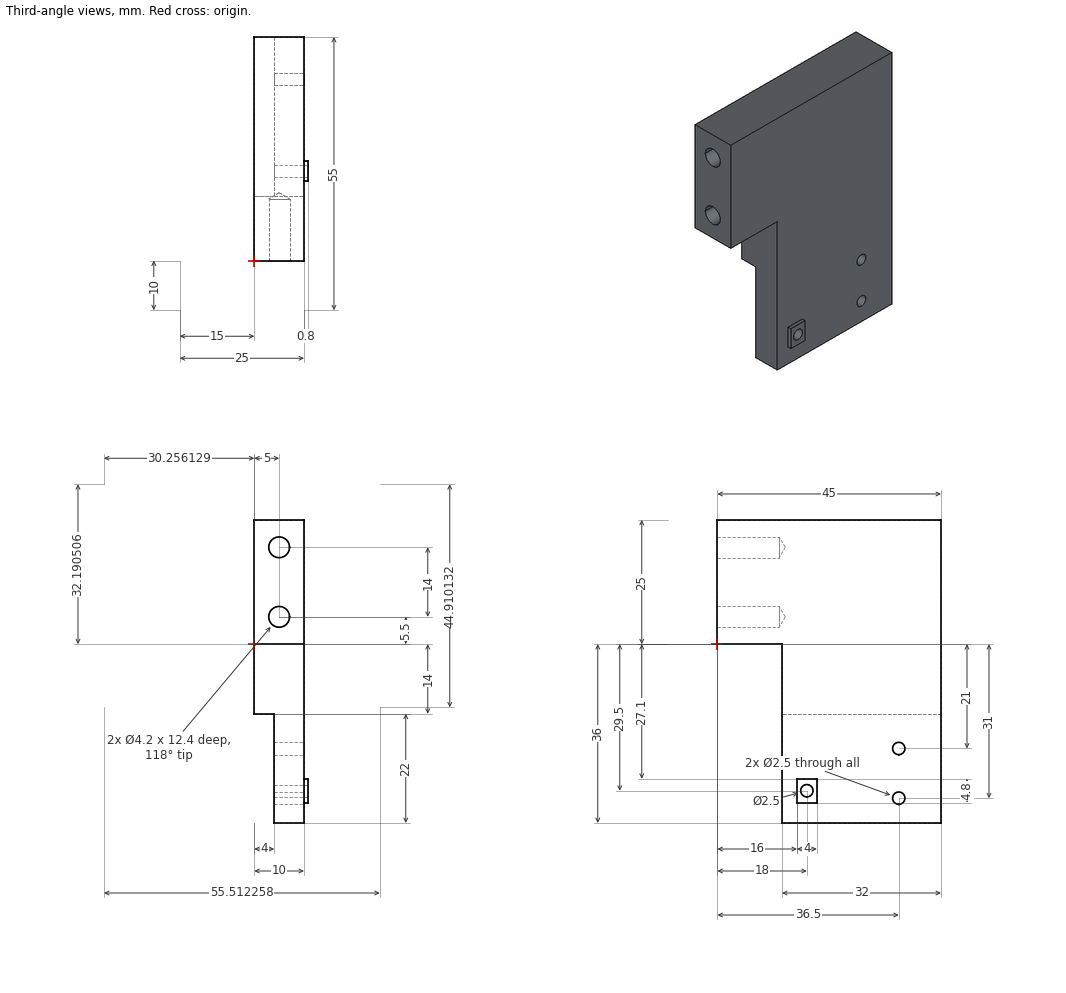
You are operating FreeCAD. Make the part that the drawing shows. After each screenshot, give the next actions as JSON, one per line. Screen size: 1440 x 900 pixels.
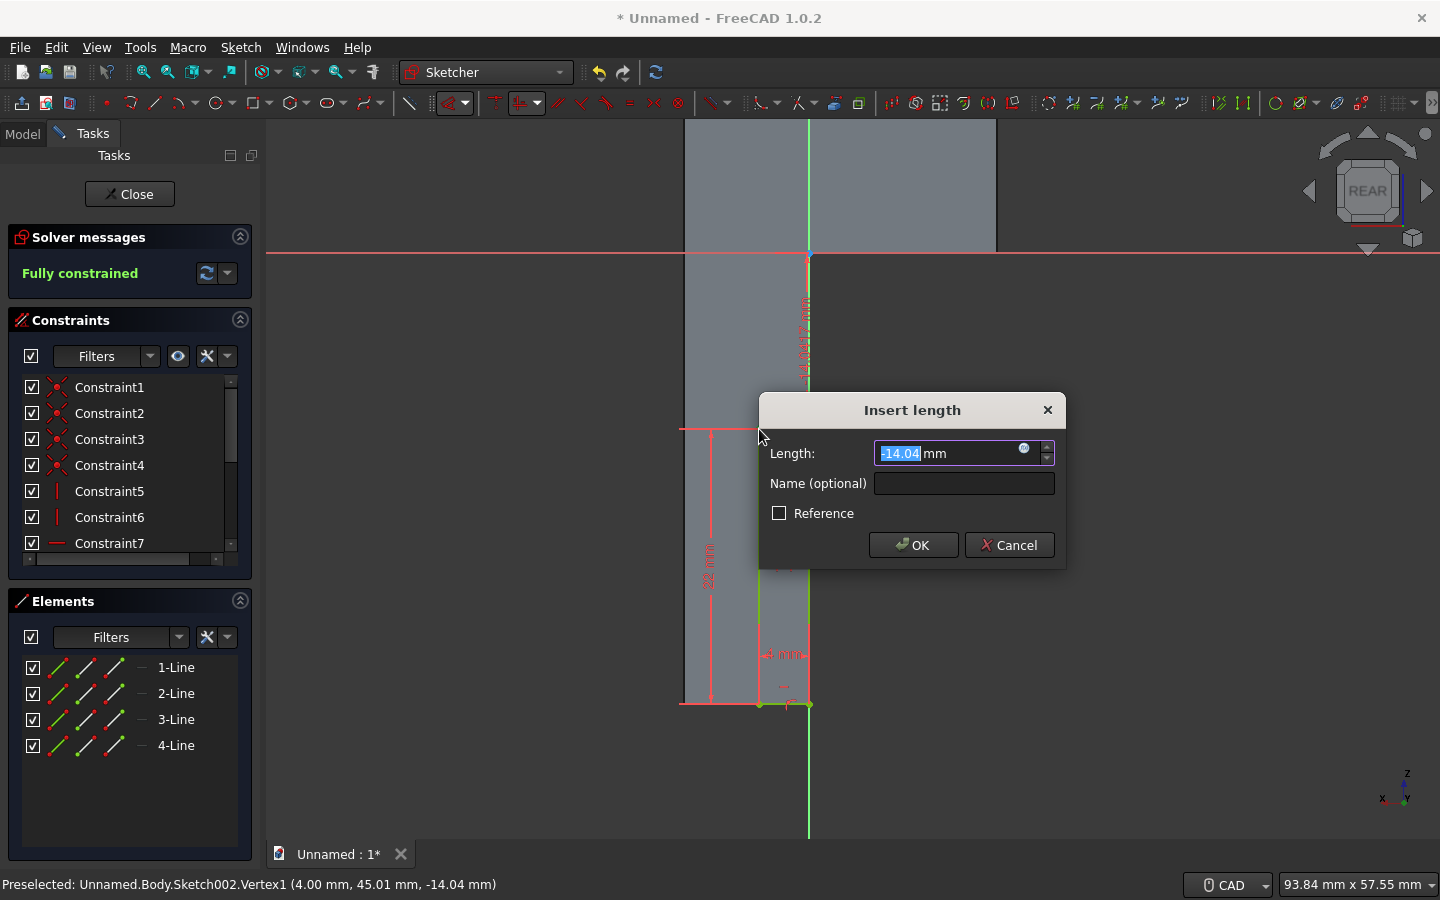
{"action": "type", "text": "-14"}
{"action": "key", "text": "Return"}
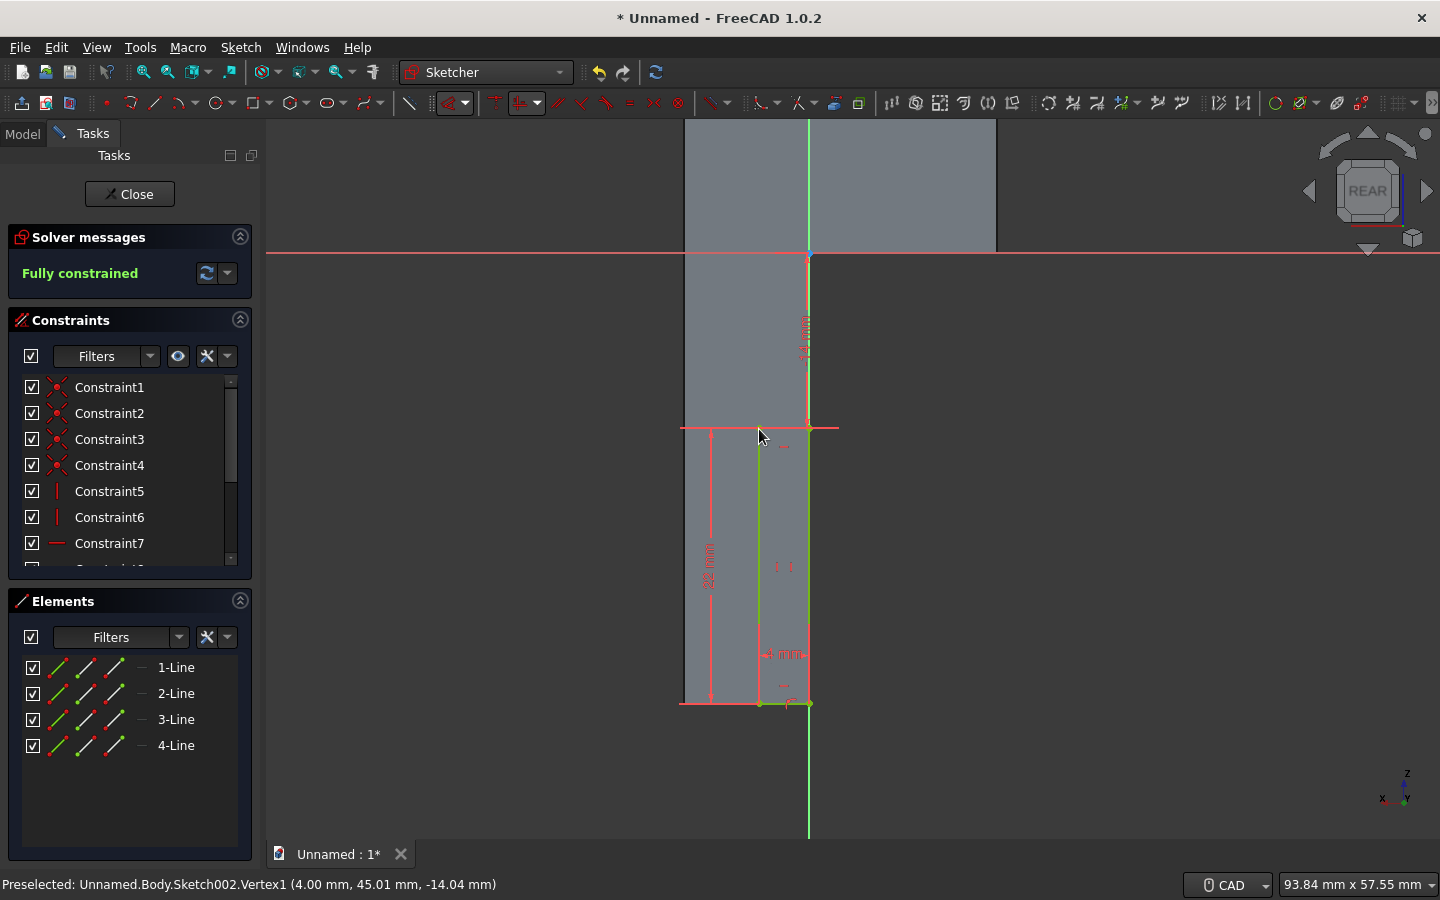
{"action": "left_click", "coordinate": [130, 194]}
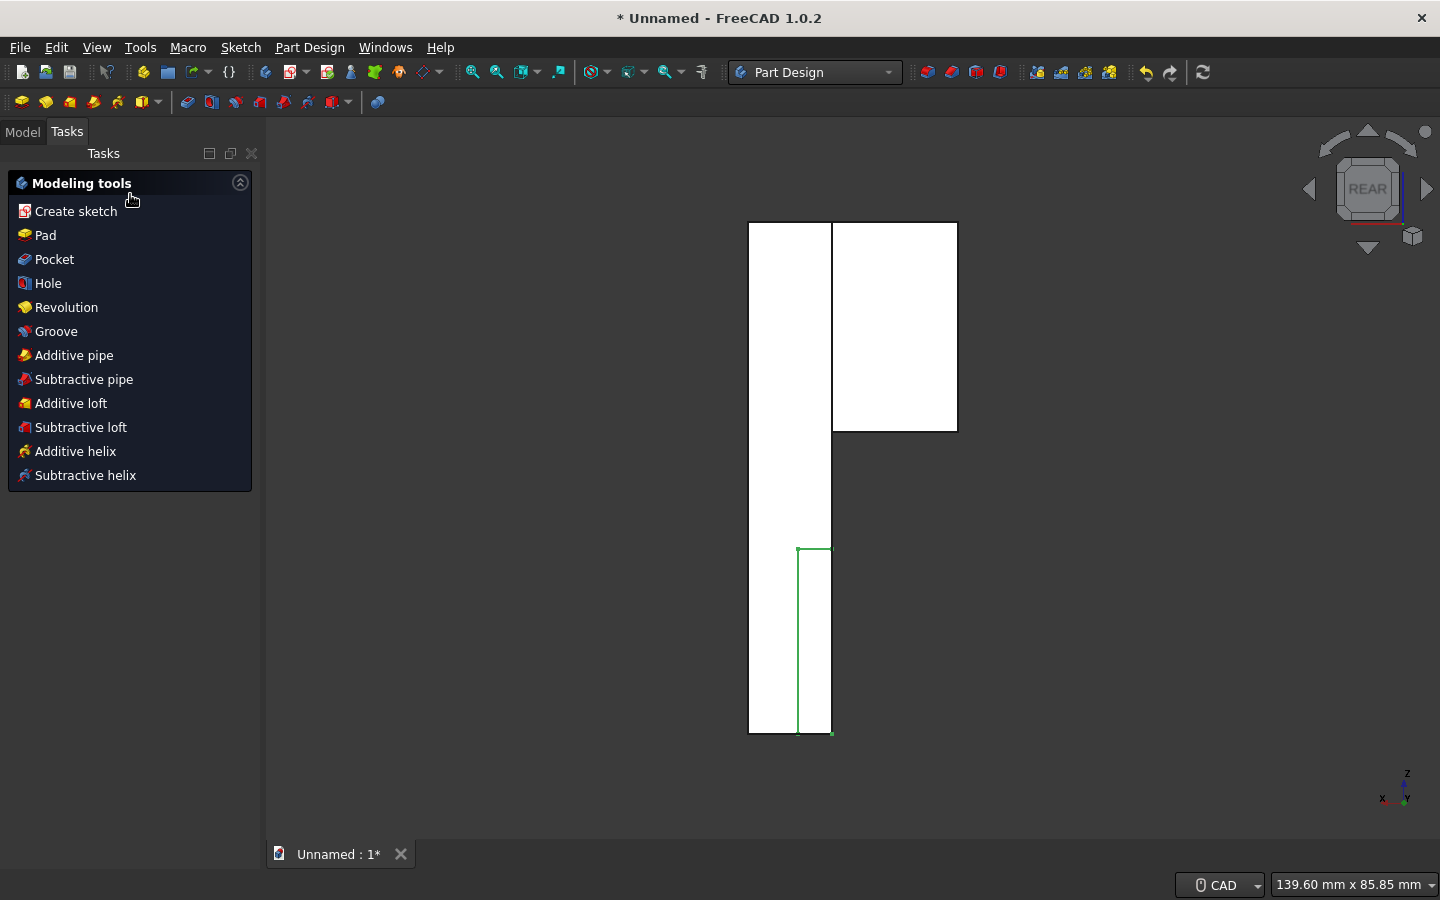
{"action": "left_click", "coordinate": [188, 102]}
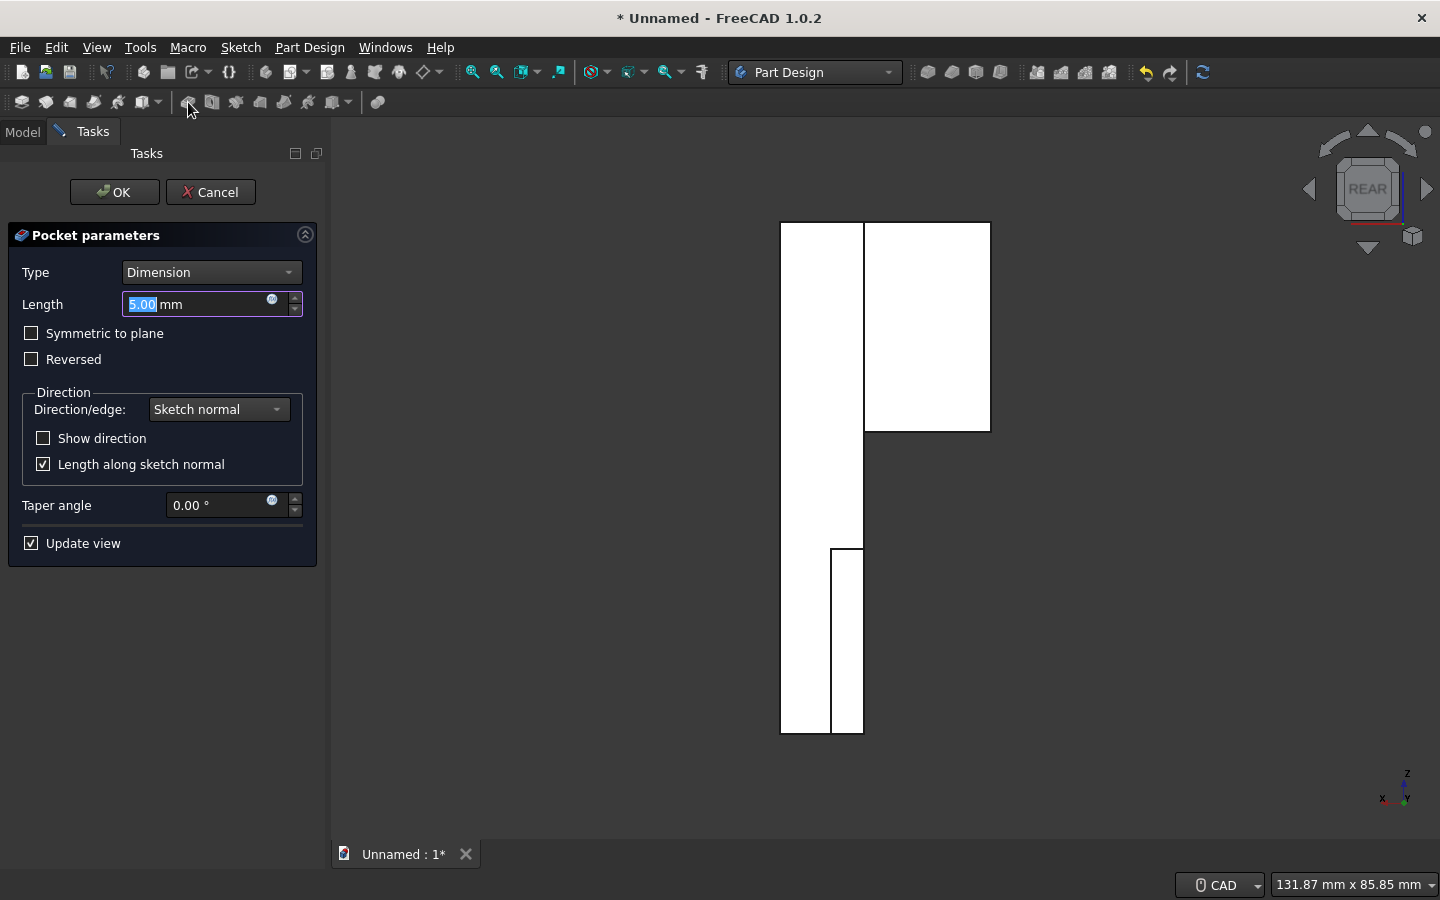
{"action": "left_click", "coordinate": [212, 272]}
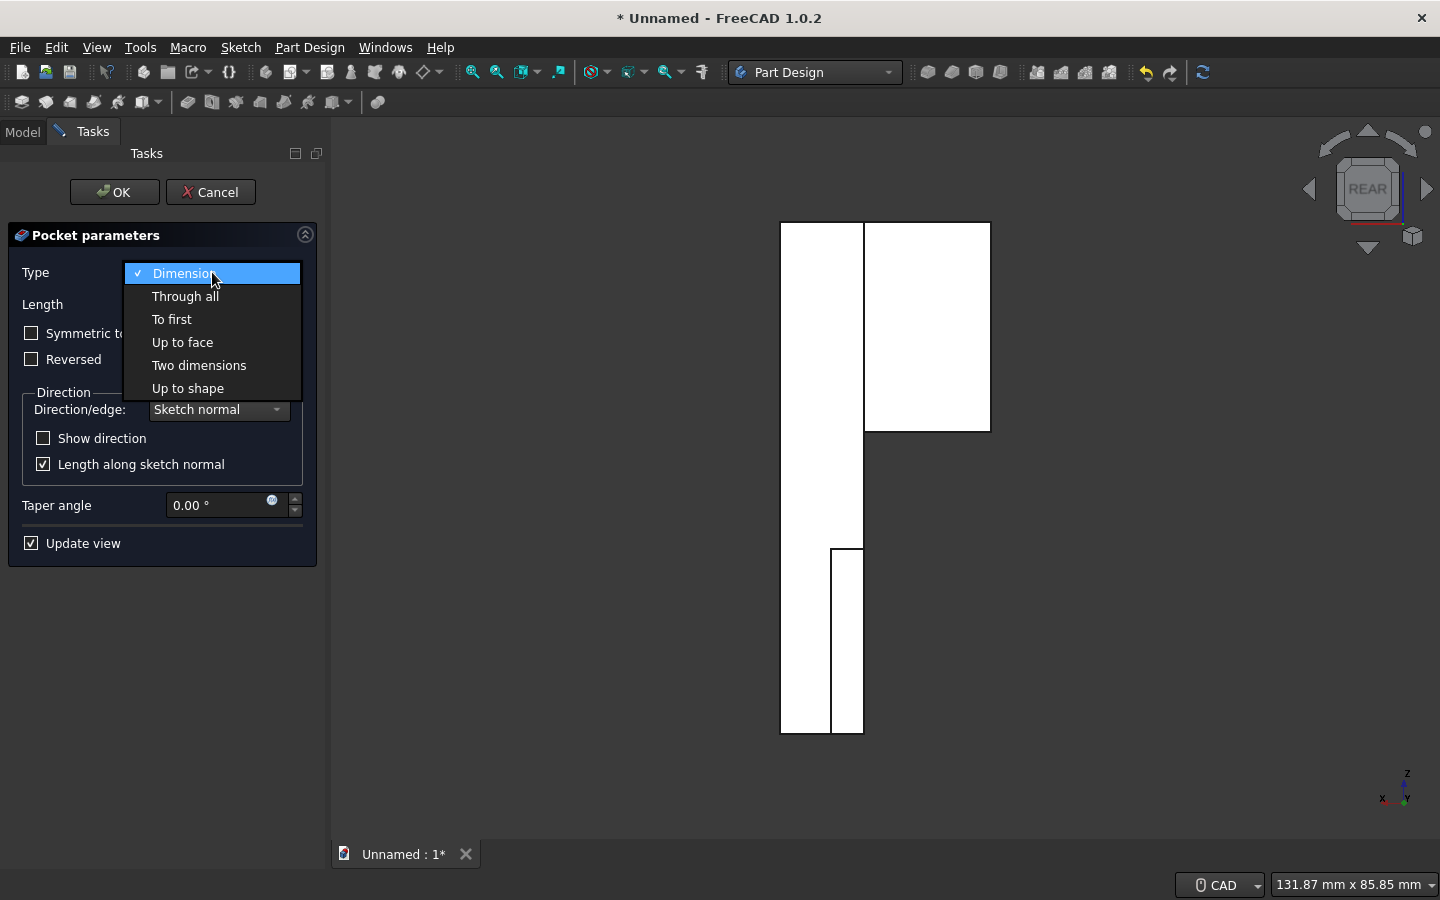
{"action": "left_click", "coordinate": [212, 296]}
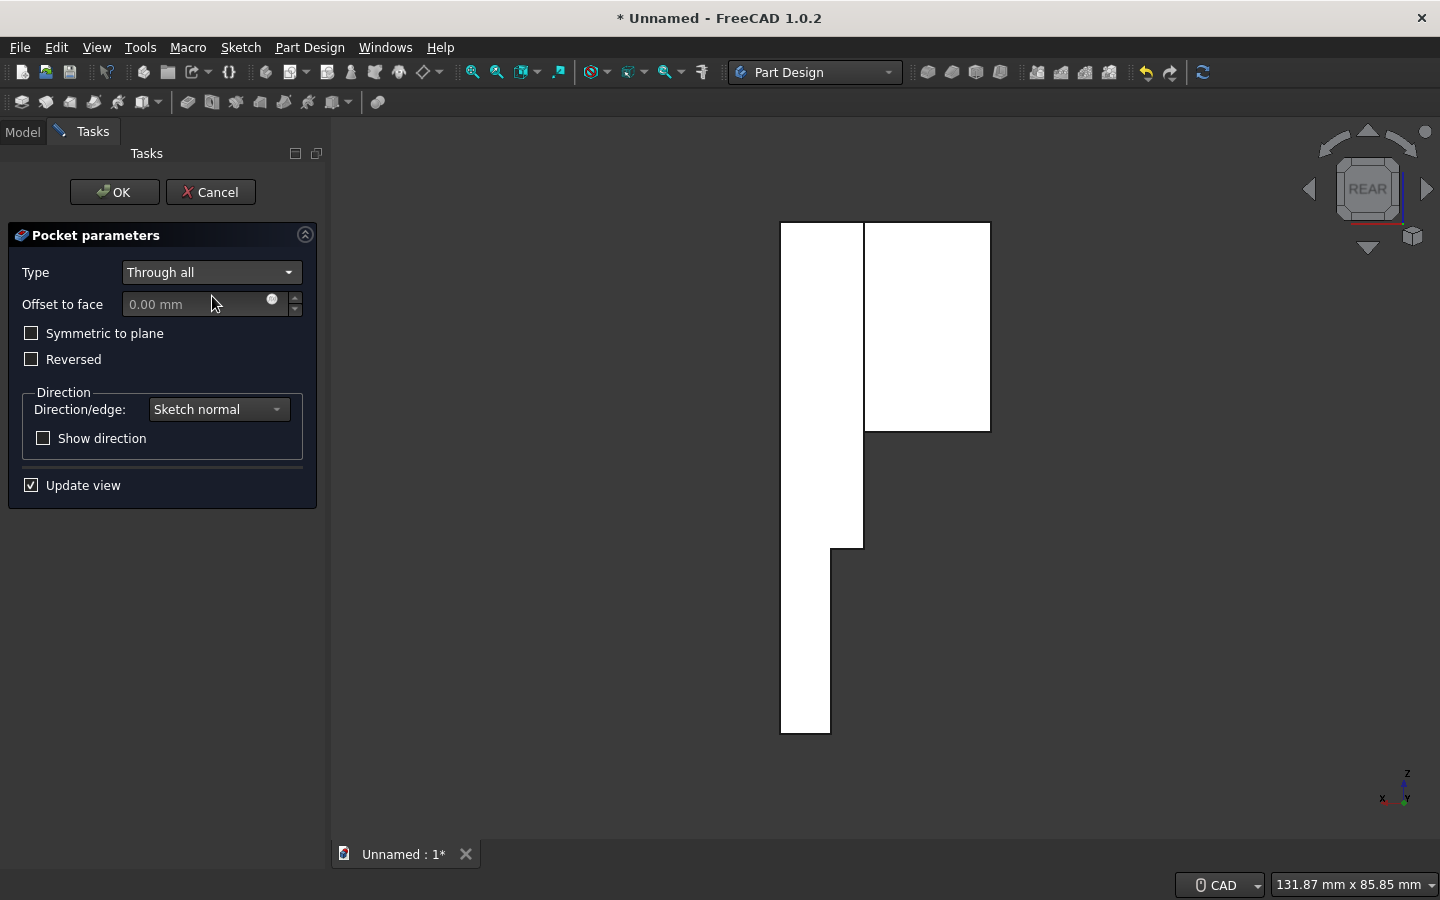
{"action": "left_click", "coordinate": [115, 192]}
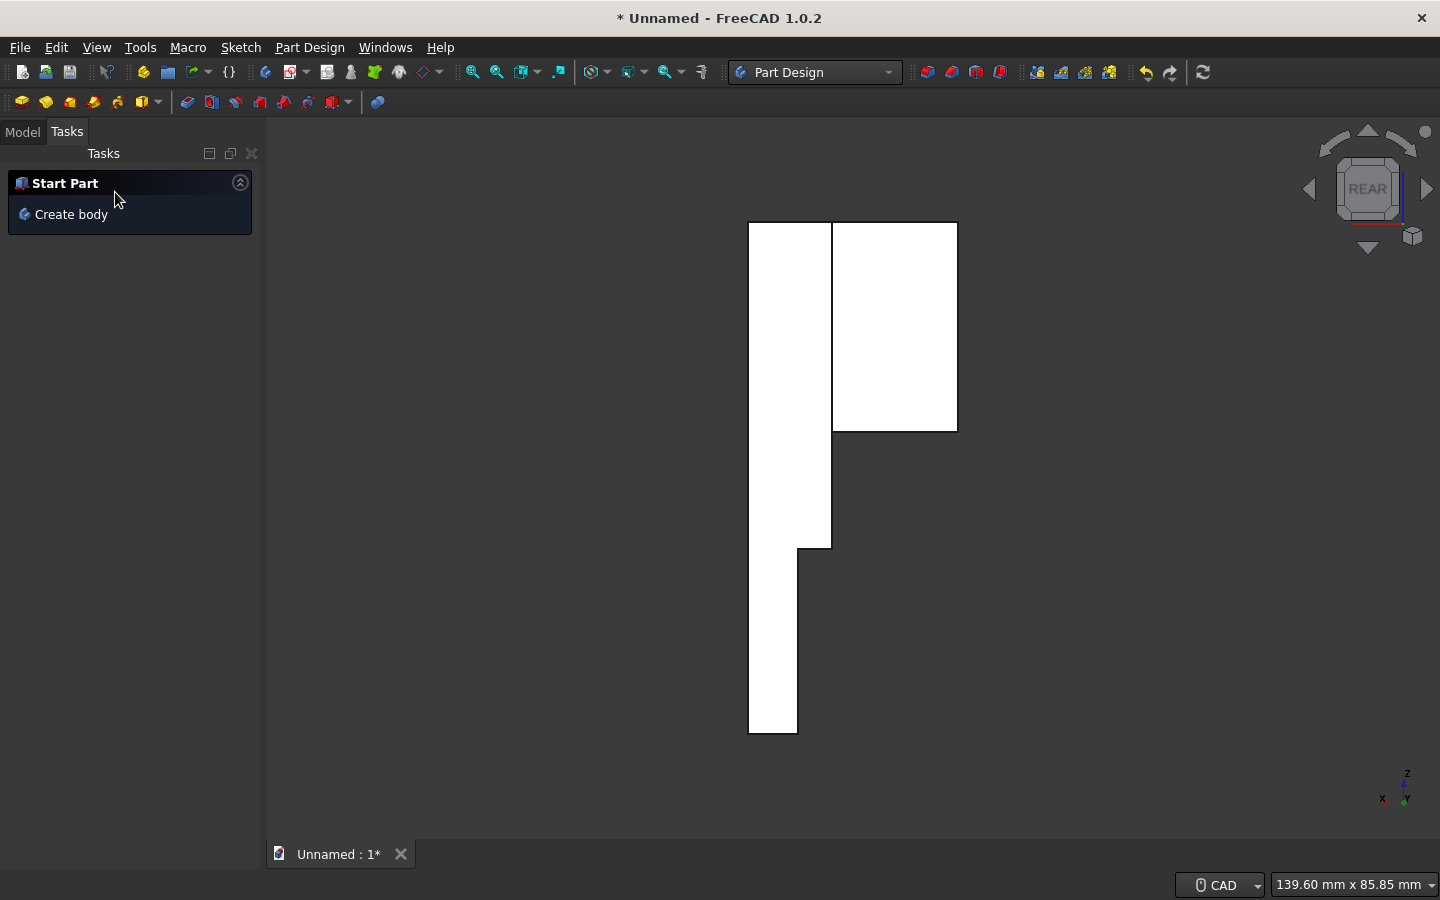
{"action": "key", "text": "0"}